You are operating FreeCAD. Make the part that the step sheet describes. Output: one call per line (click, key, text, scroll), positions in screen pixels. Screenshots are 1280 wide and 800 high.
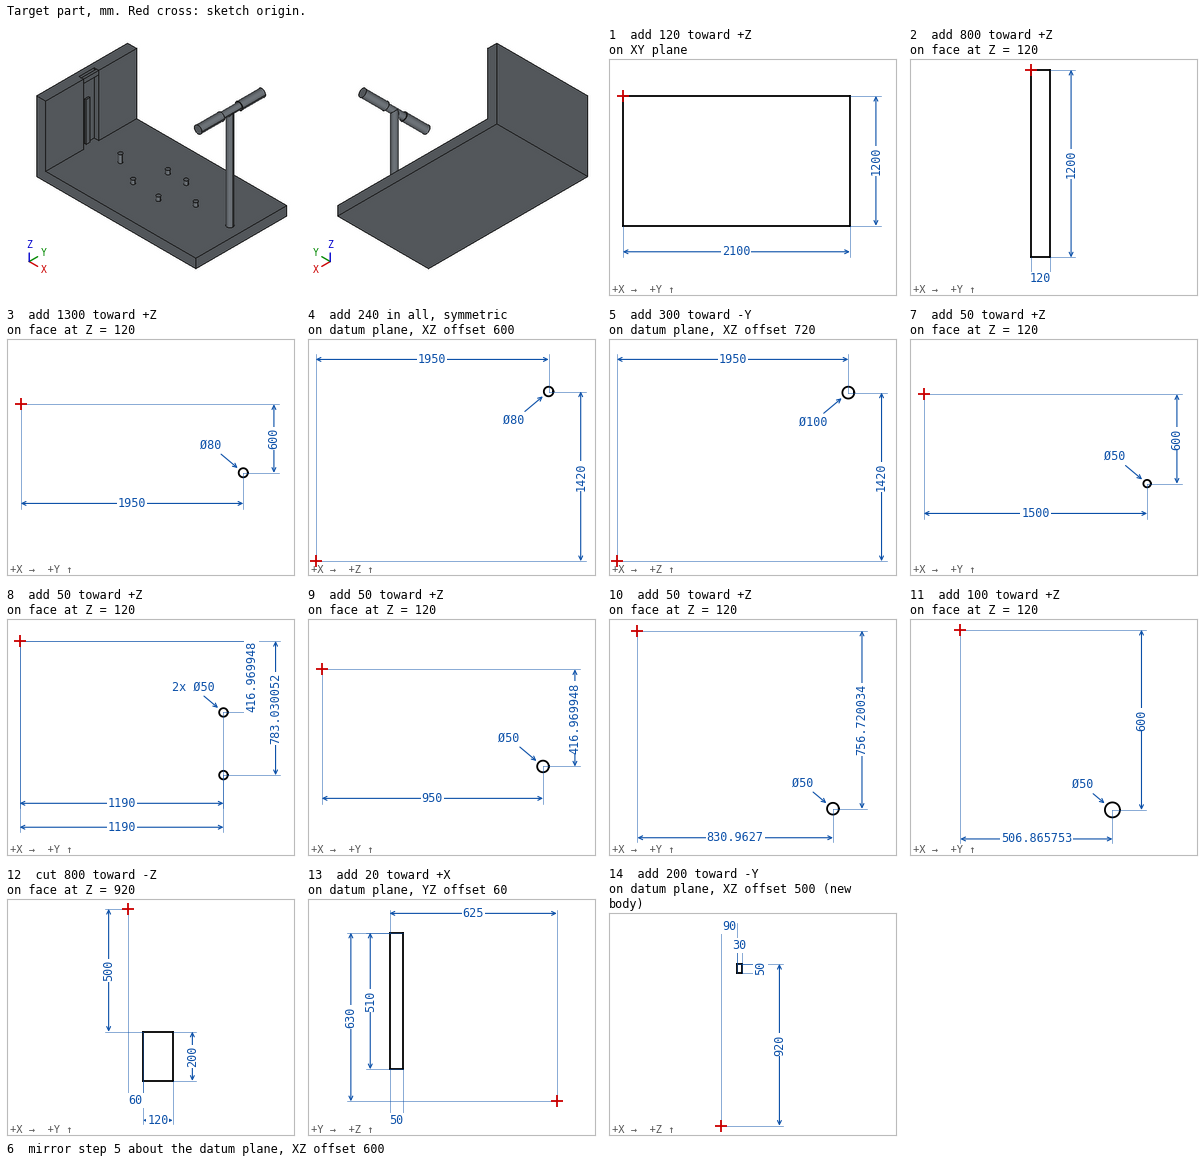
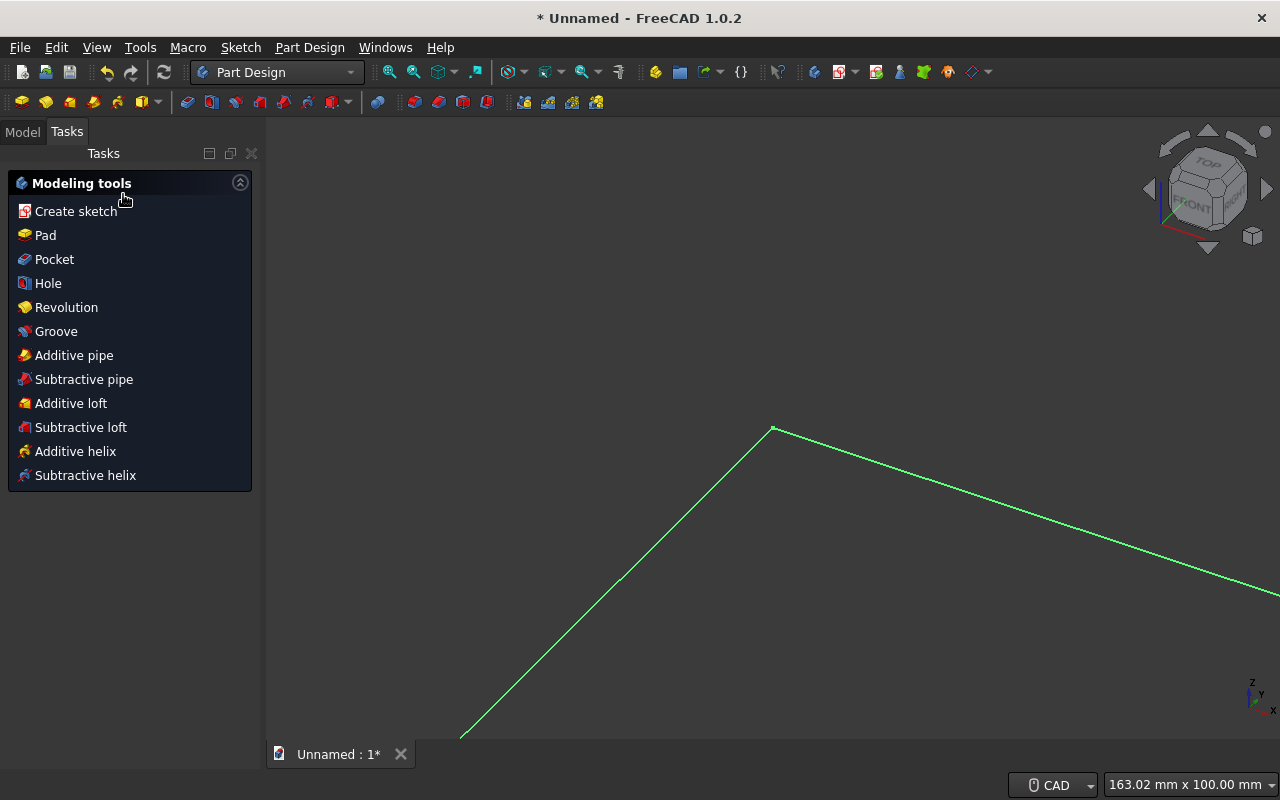
click(22, 102)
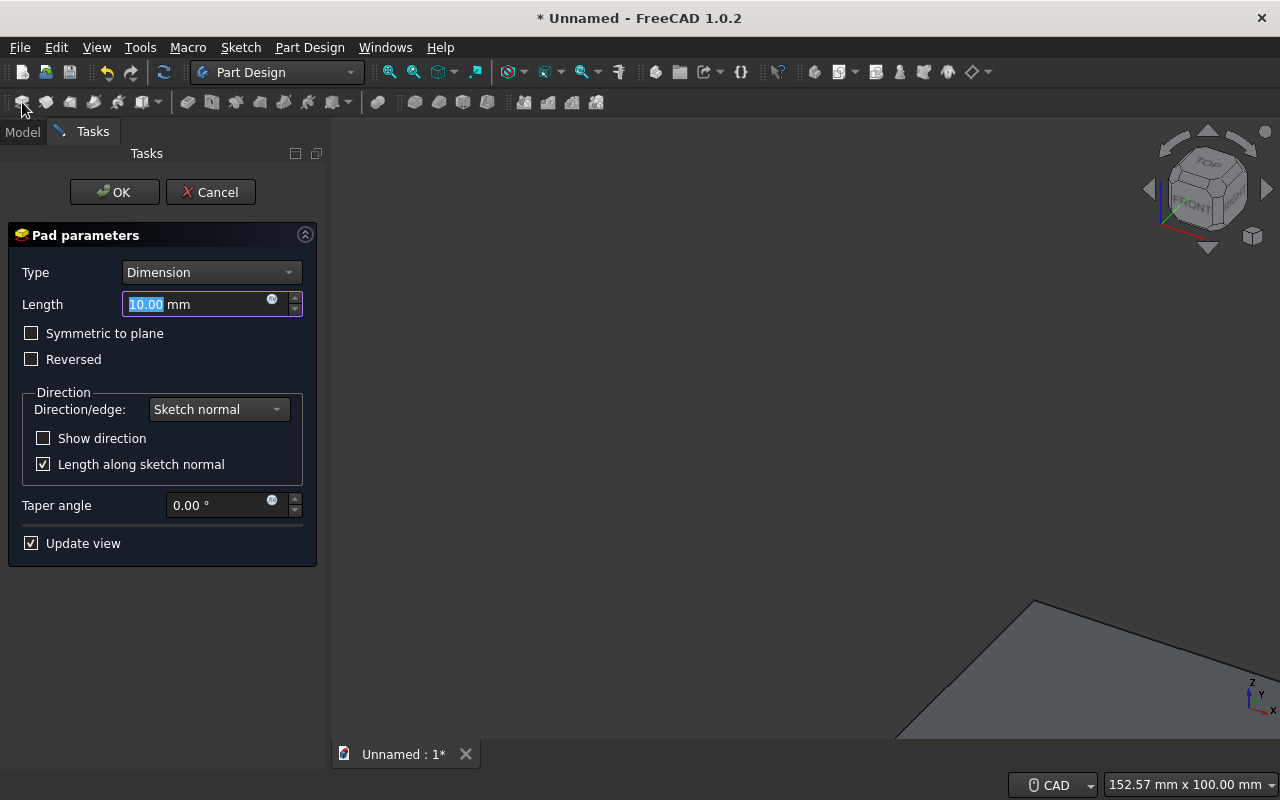
text(120)
key(Tab)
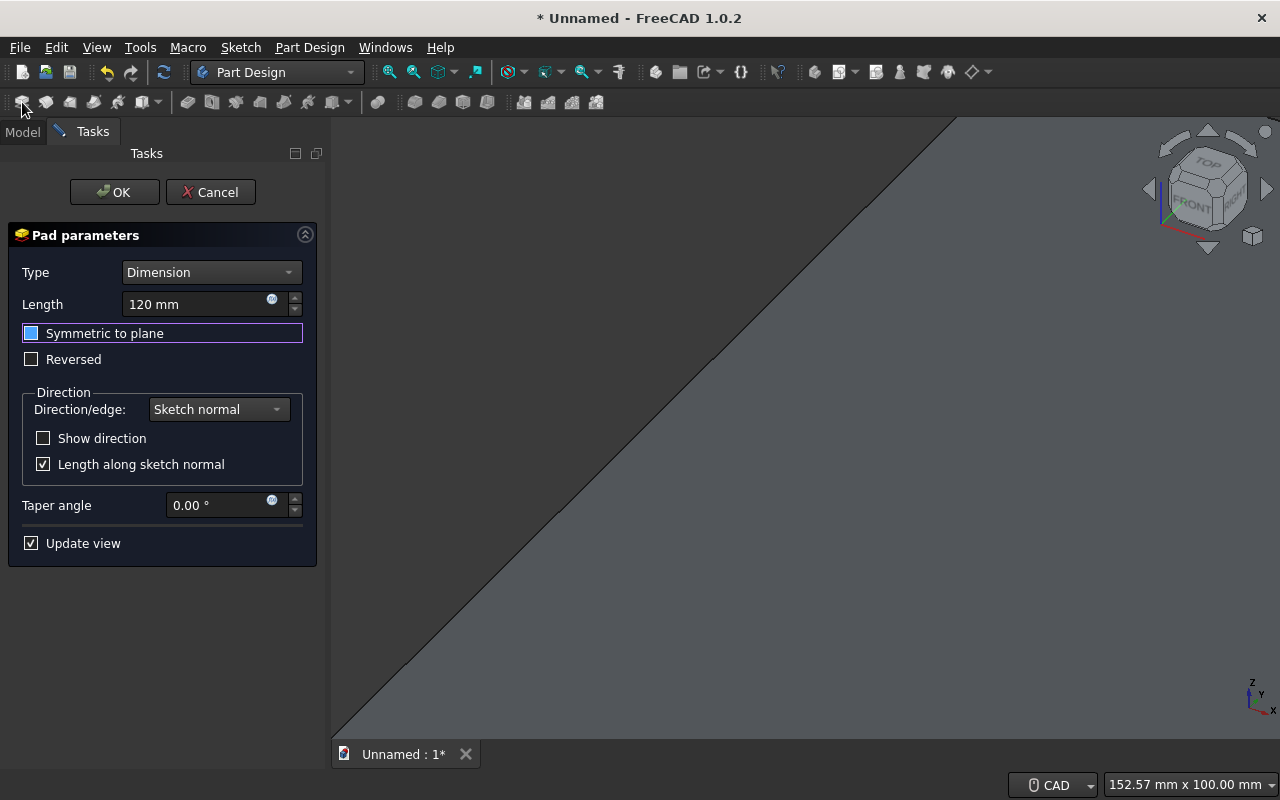
click(115, 192)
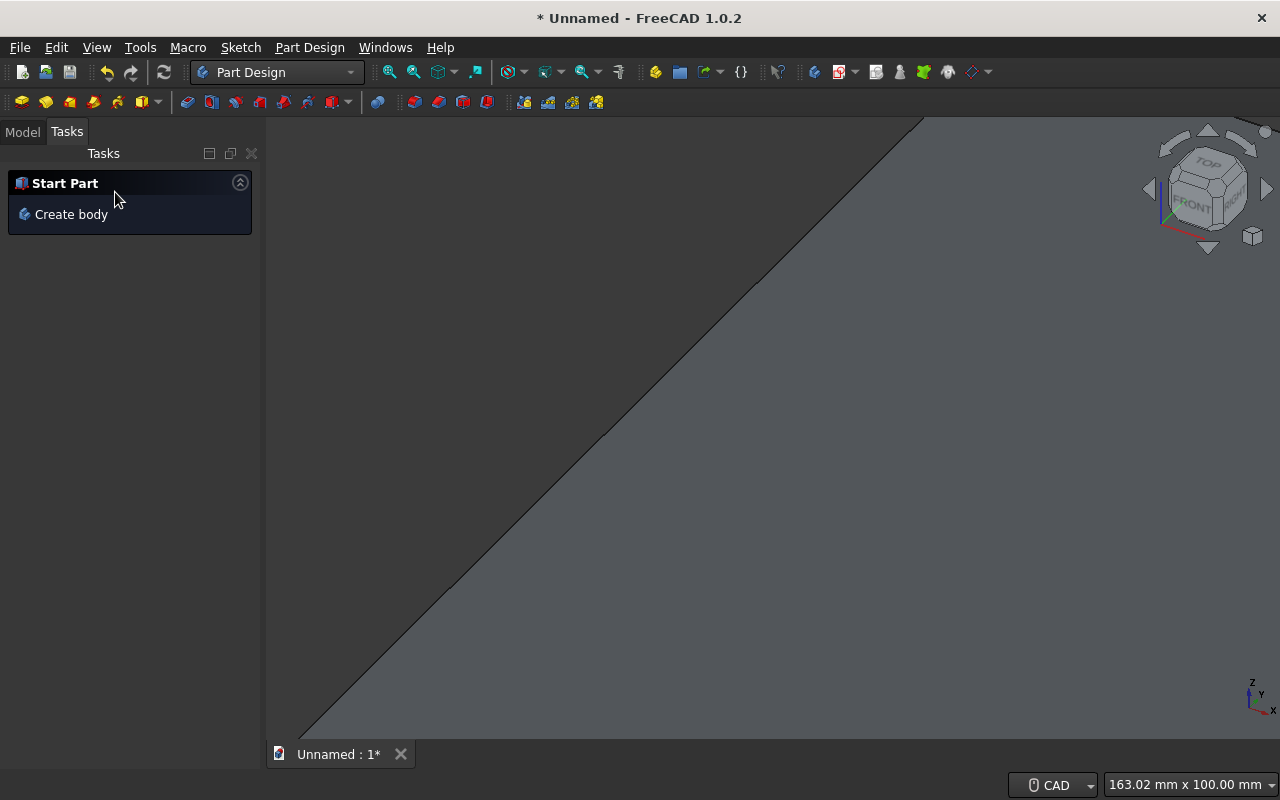
click(390, 72)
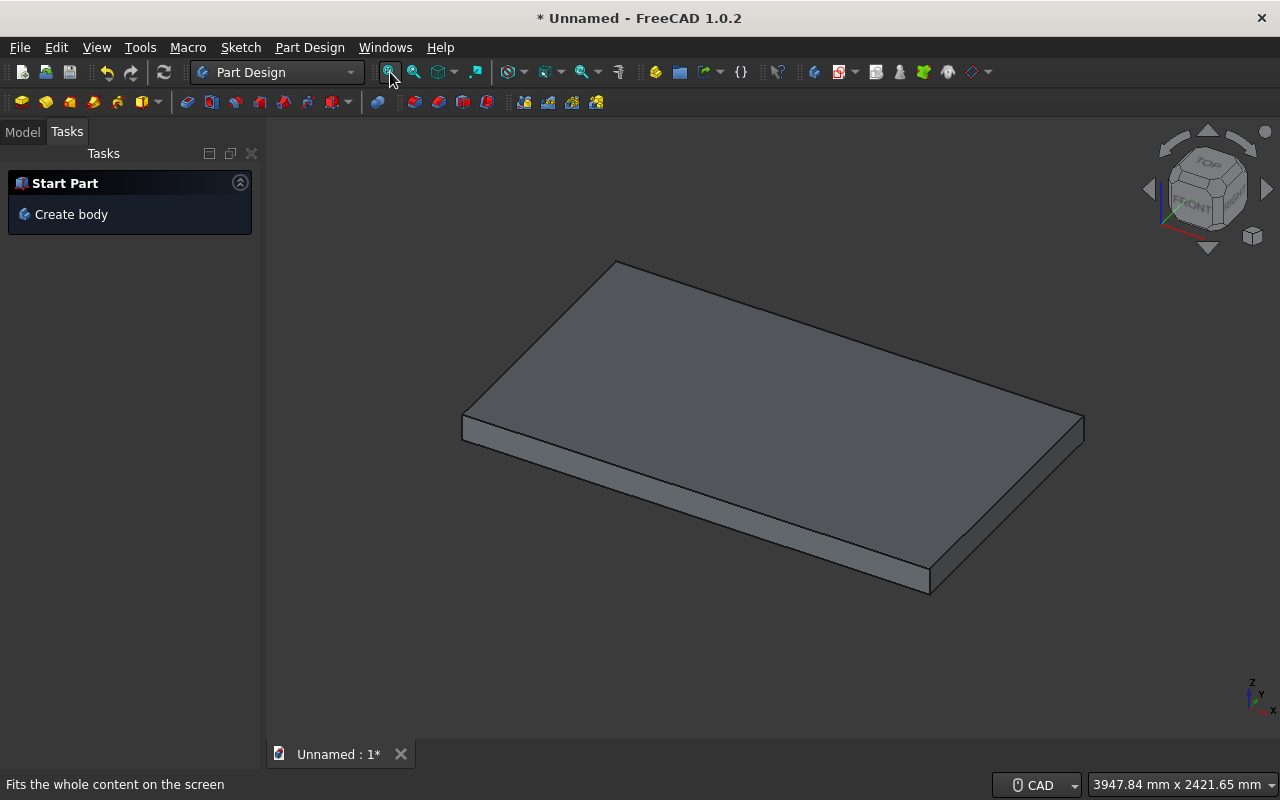
click(840, 436)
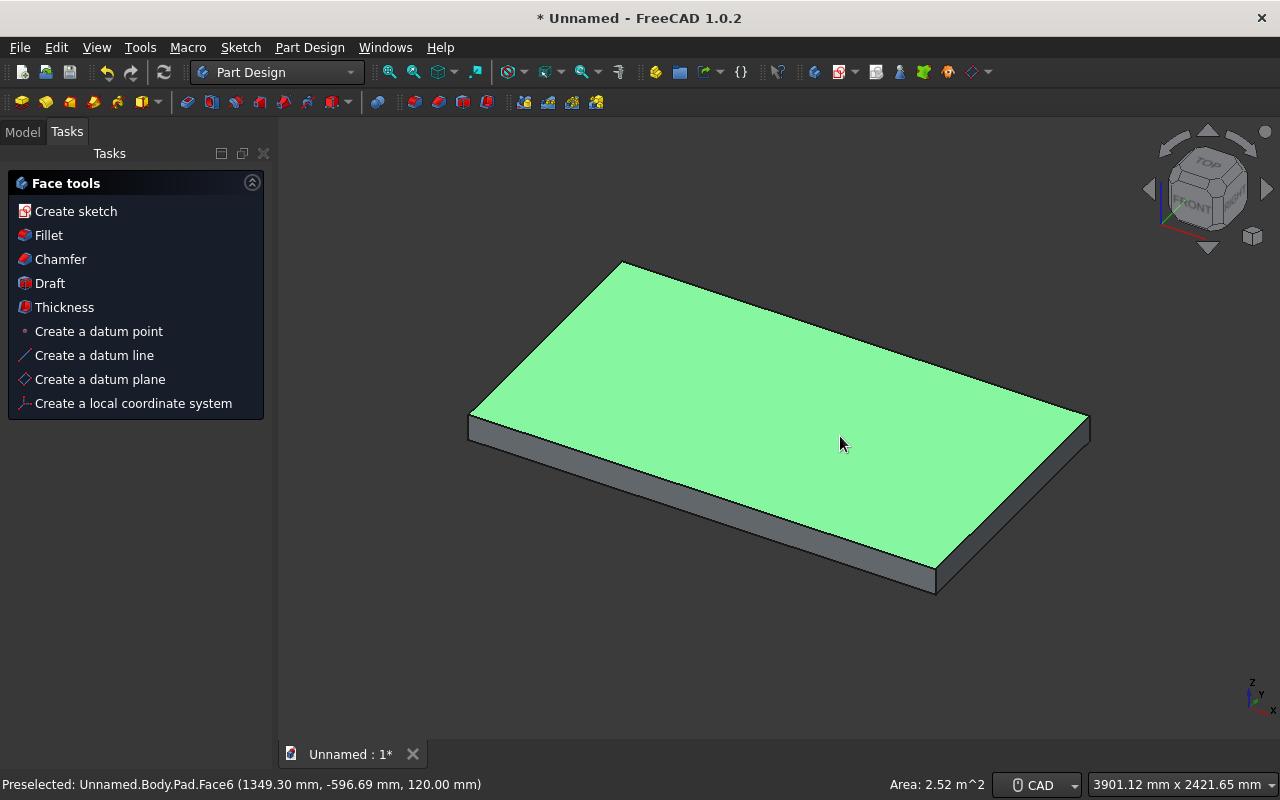
click(840, 72)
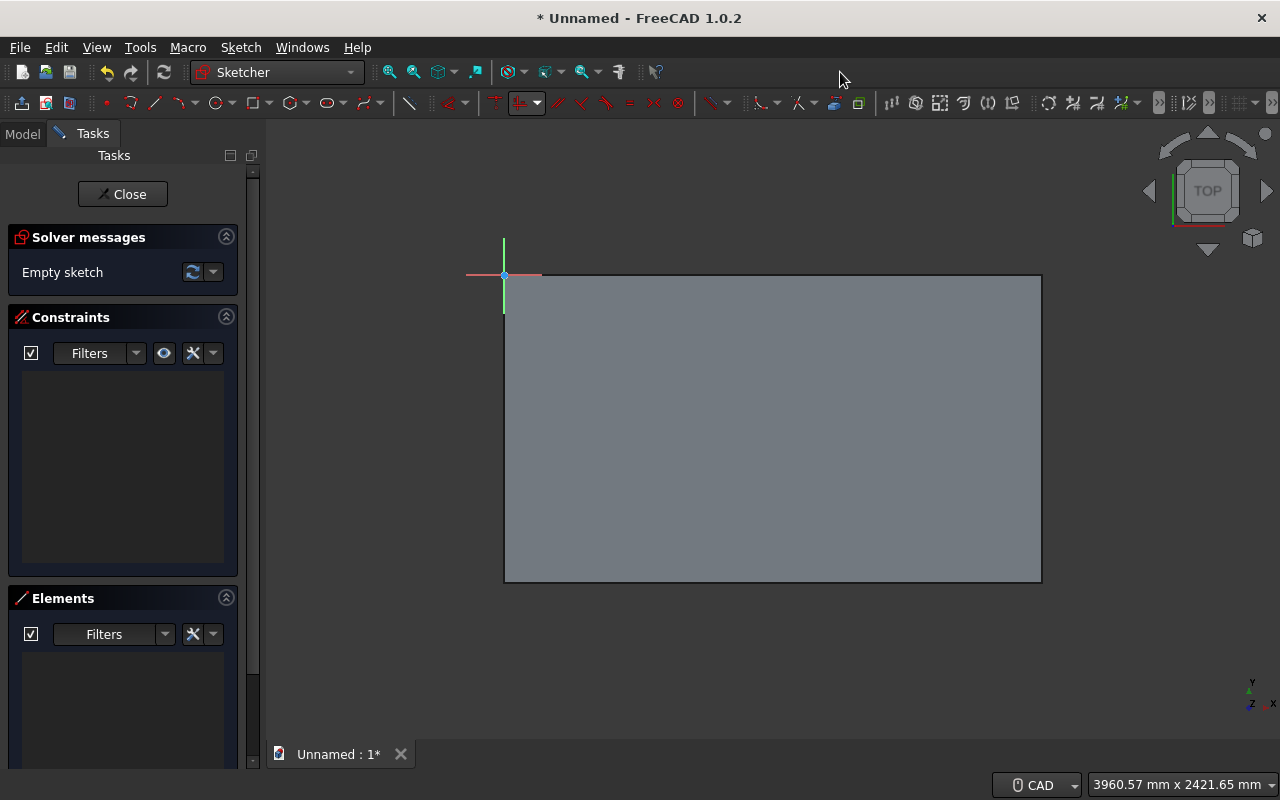
click(254, 104)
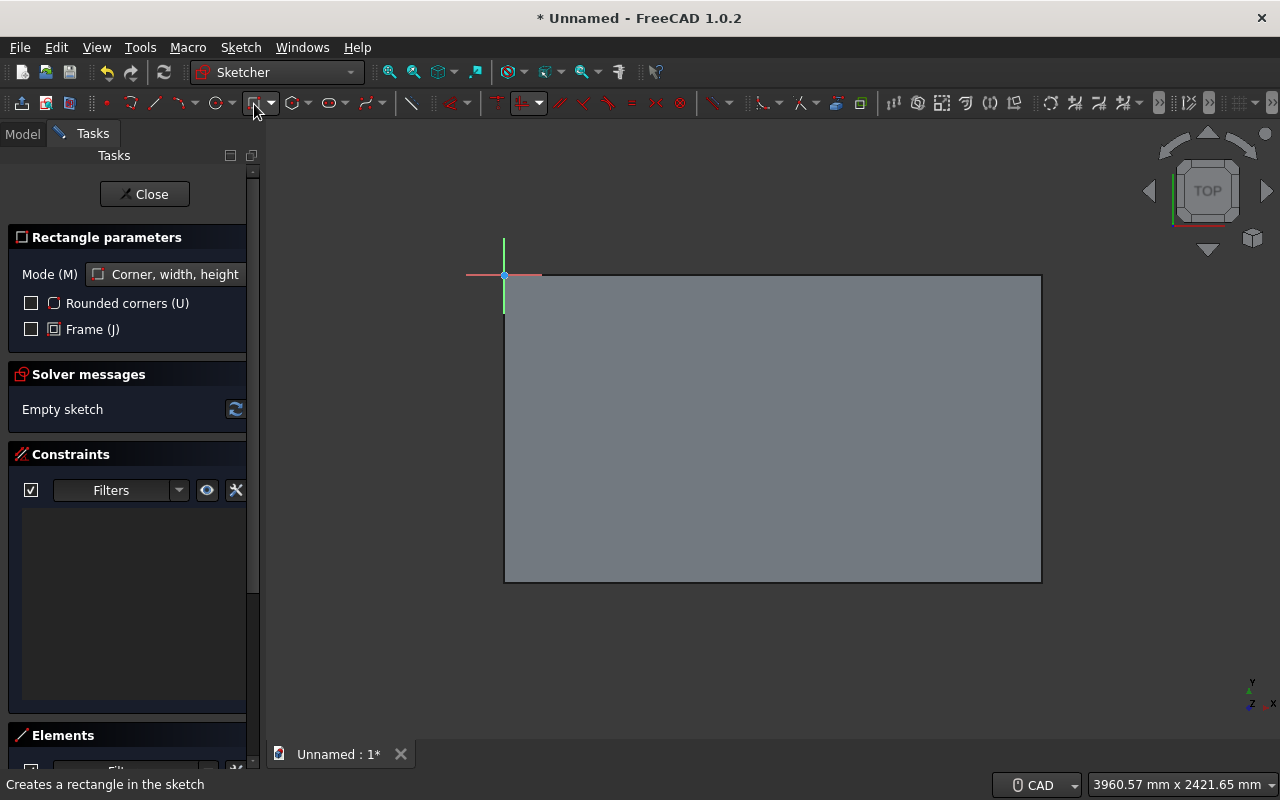
click(504, 275)
move(535, 583)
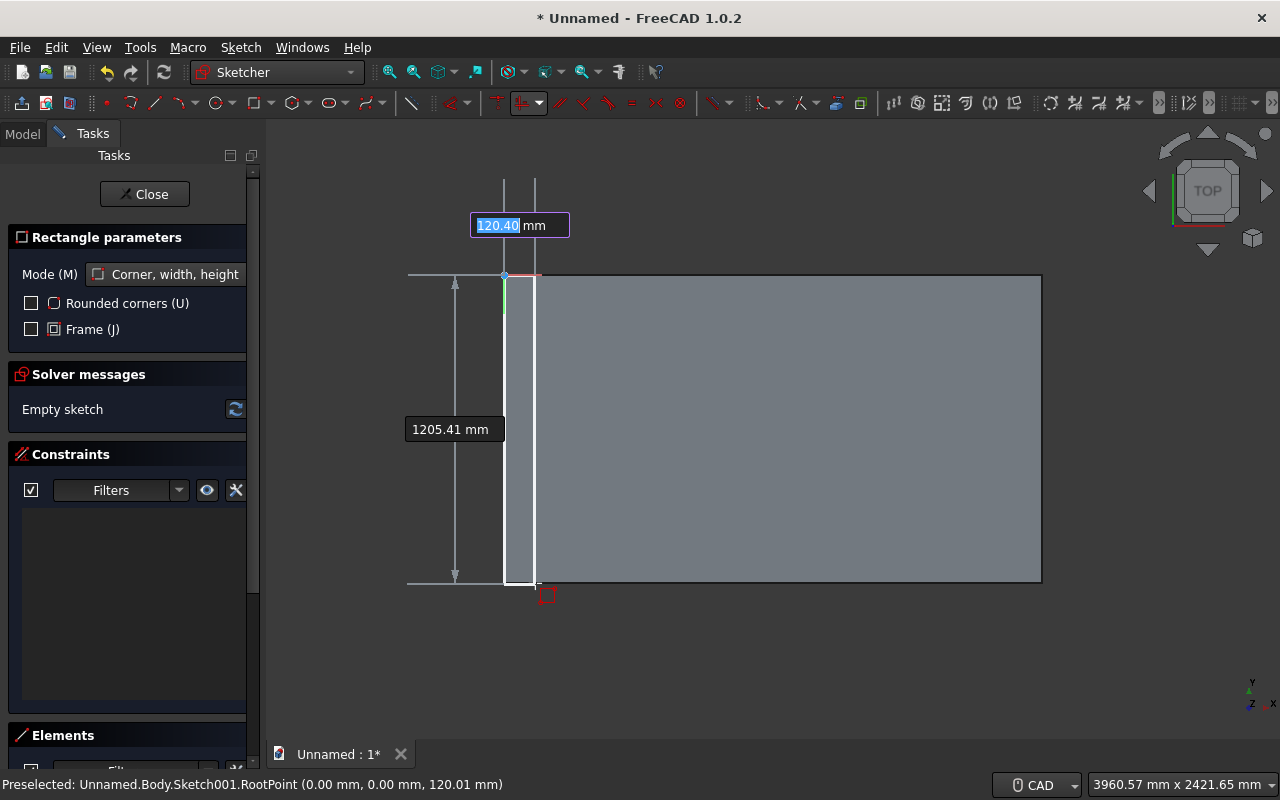
text(120)
key(Tab)
text(1200)
key(Return)
key(Escape)